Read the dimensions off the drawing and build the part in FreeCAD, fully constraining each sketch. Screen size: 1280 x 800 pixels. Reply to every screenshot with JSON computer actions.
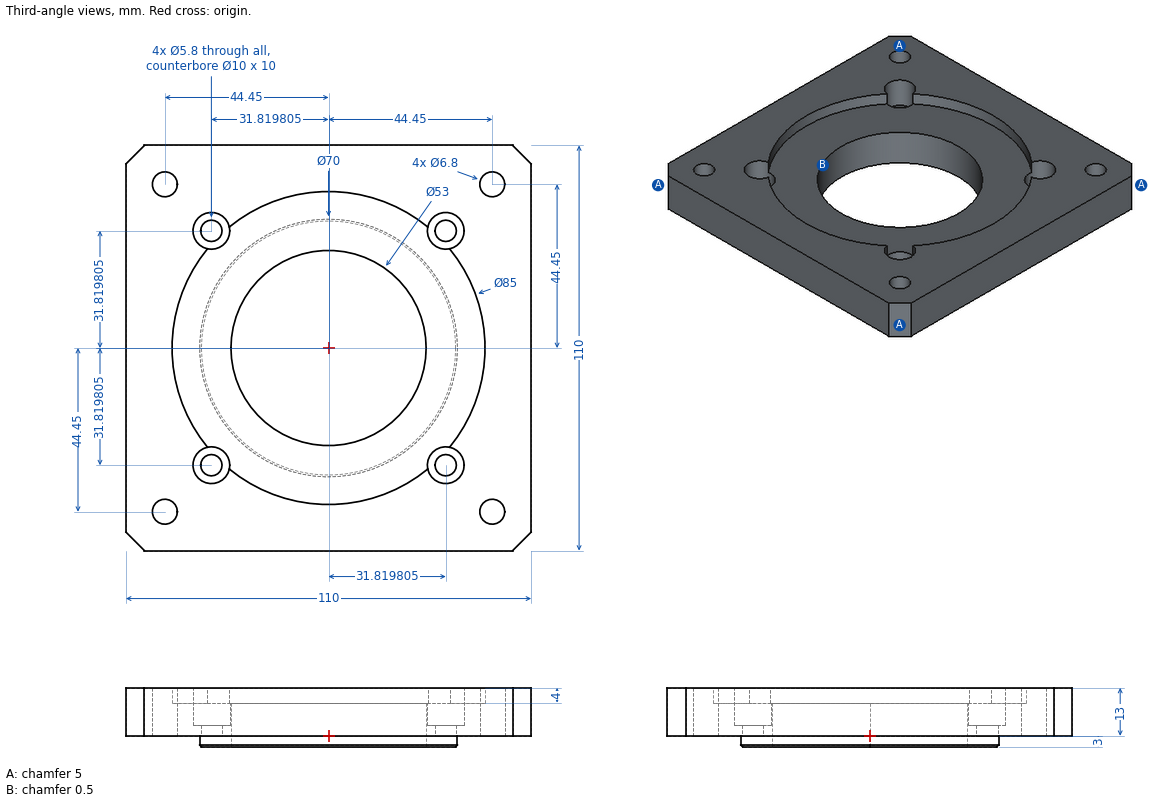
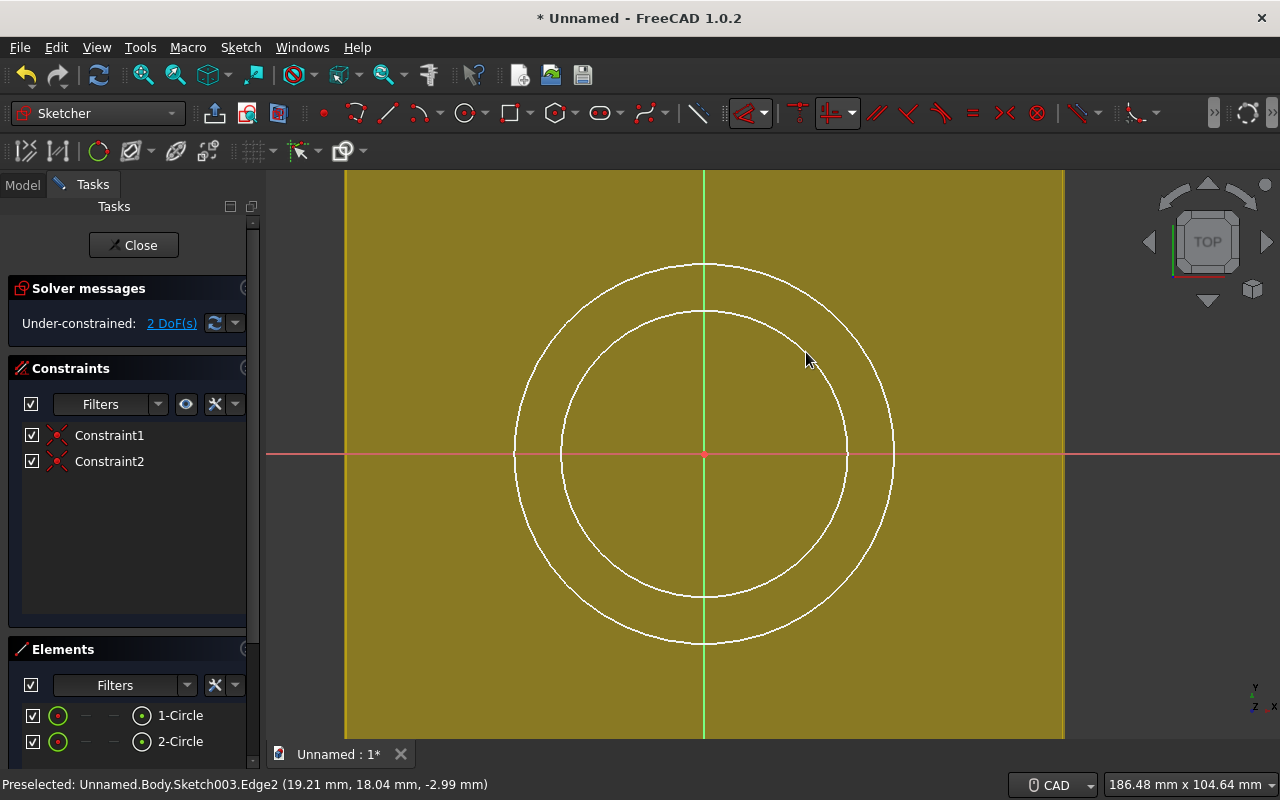
{"action": "left_click", "coordinate": [838, 319]}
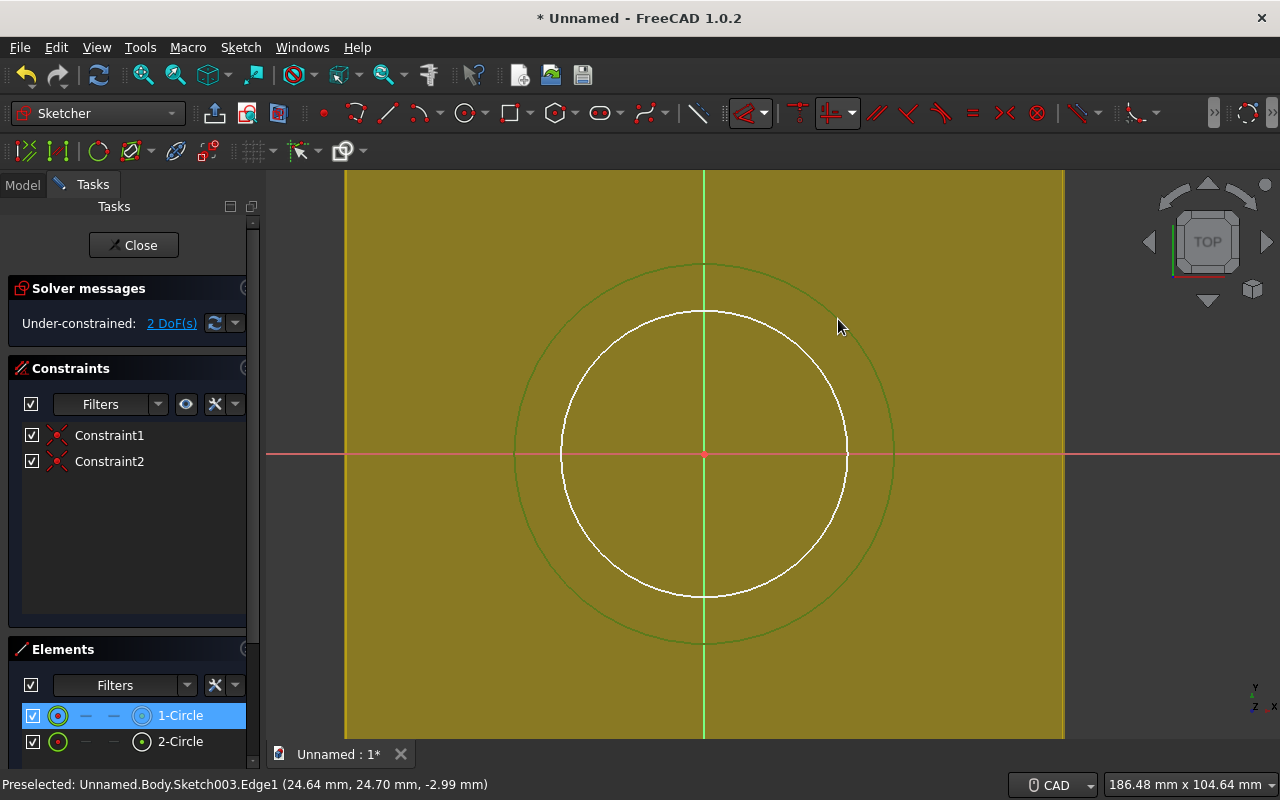
{"action": "left_click", "coordinate": [766, 114]}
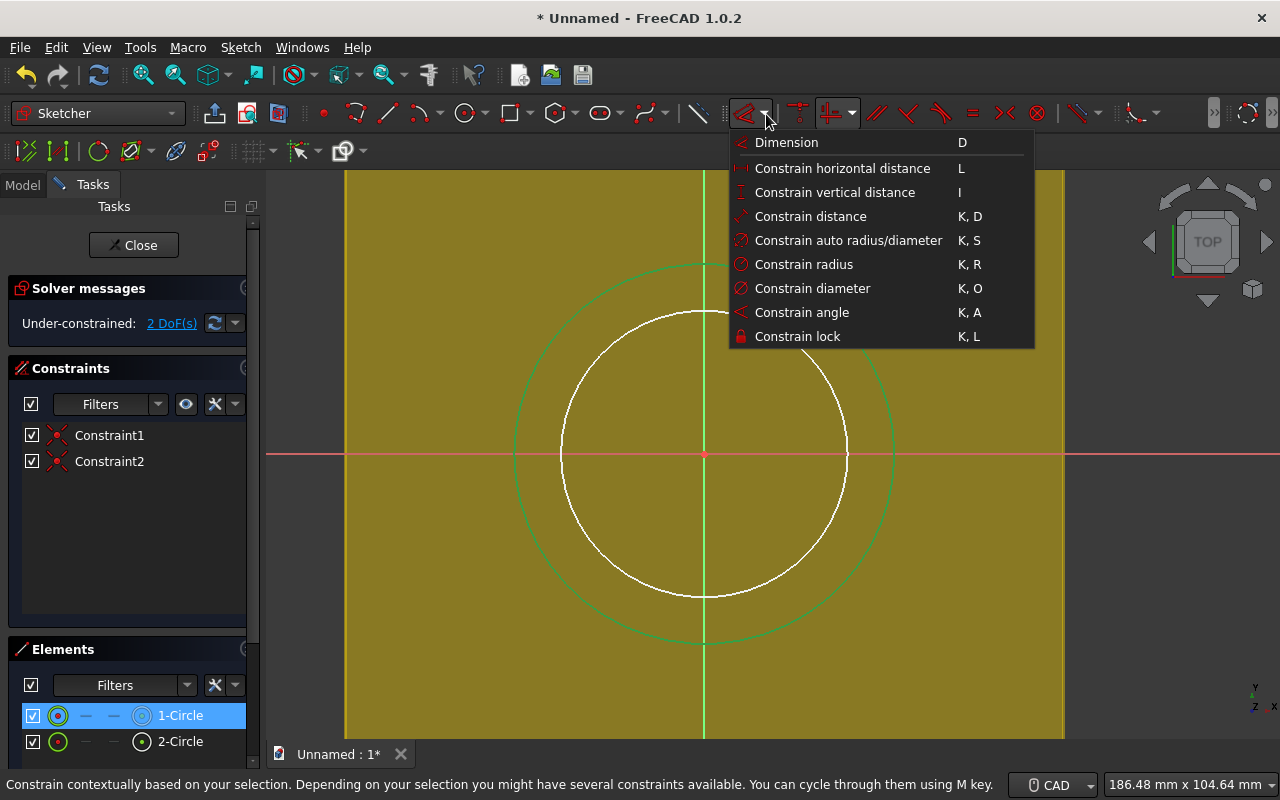
{"action": "left_click", "coordinate": [882, 288]}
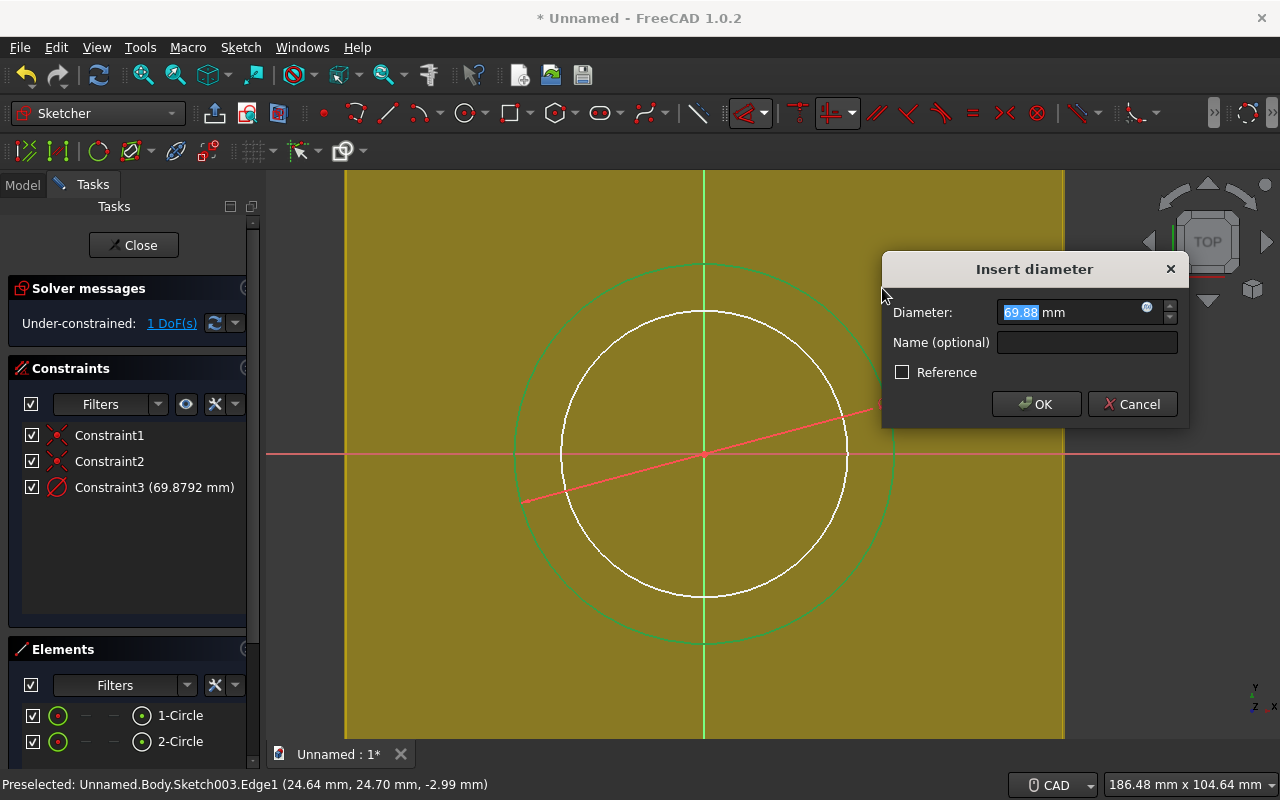
{"action": "type", "text": "70"}
{"action": "key", "text": "Return"}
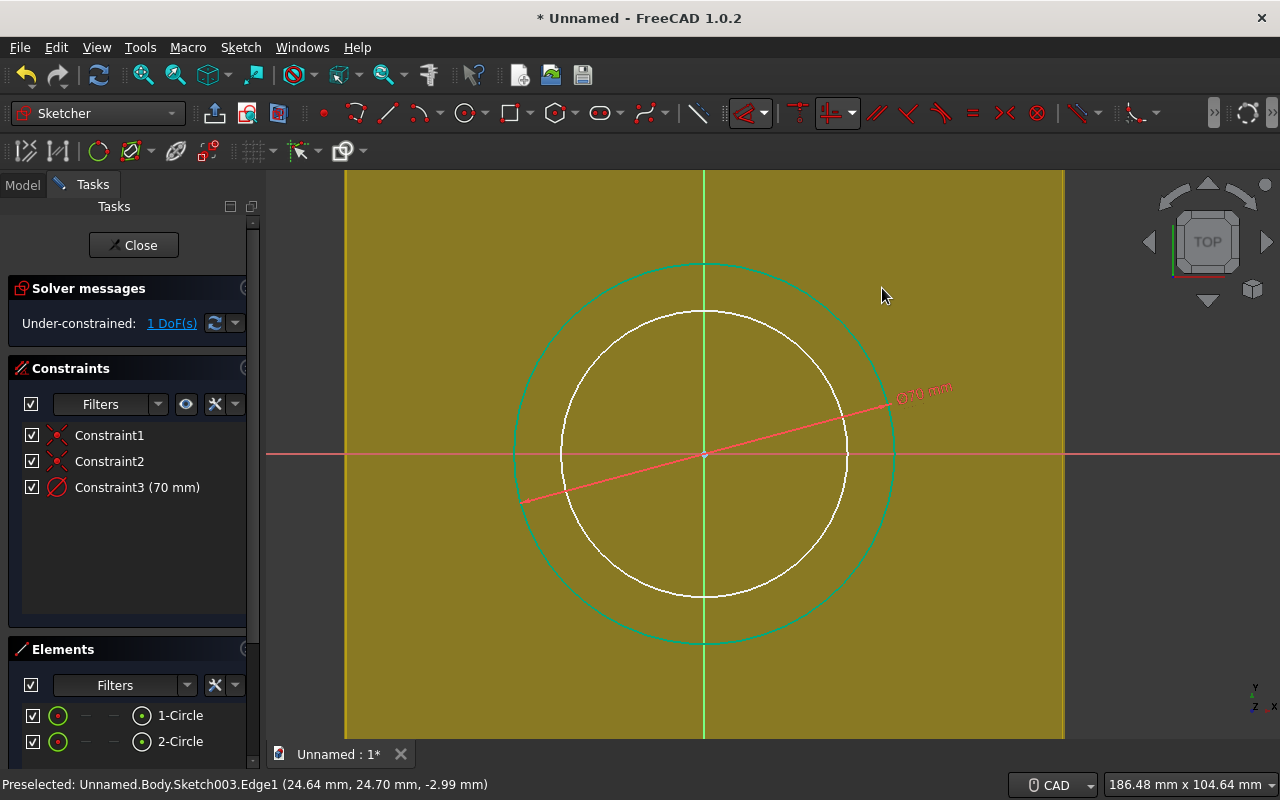
{"action": "left_click", "coordinate": [805, 352]}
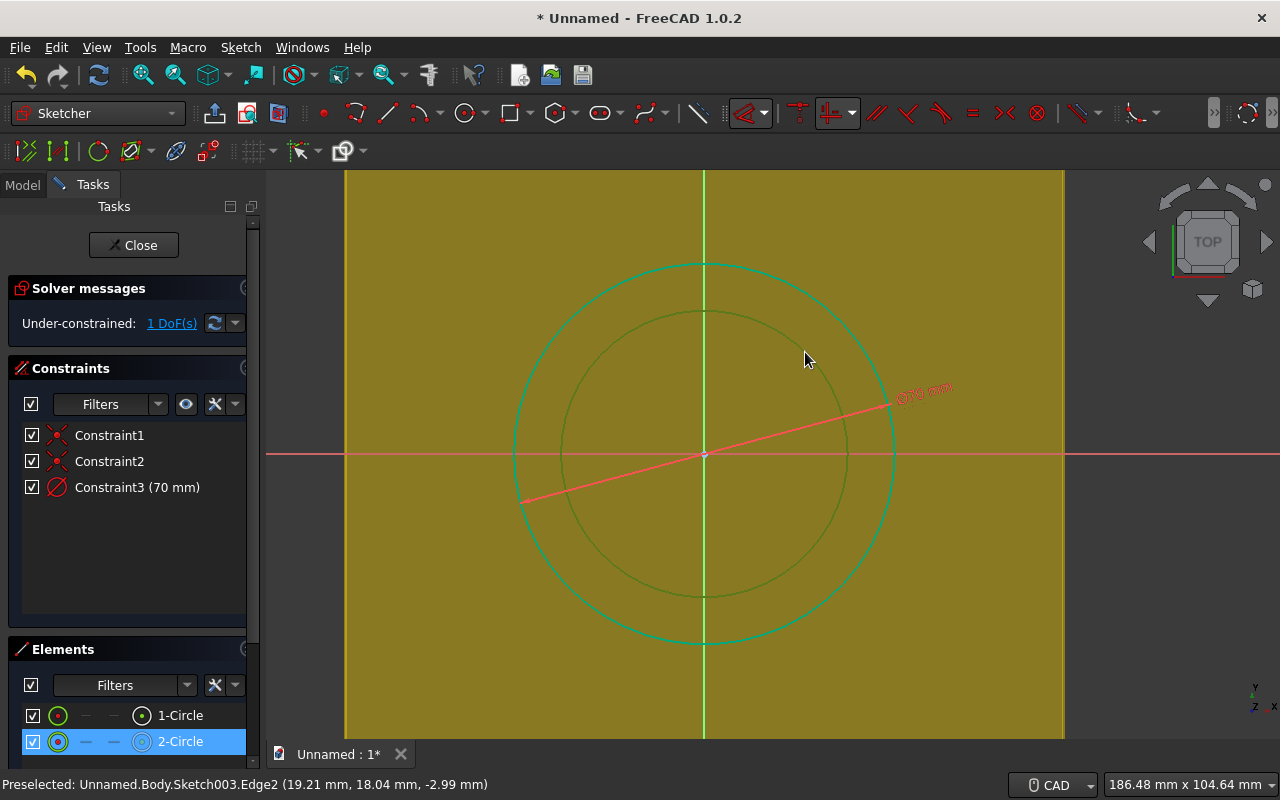
{"action": "key", "text": "k o"}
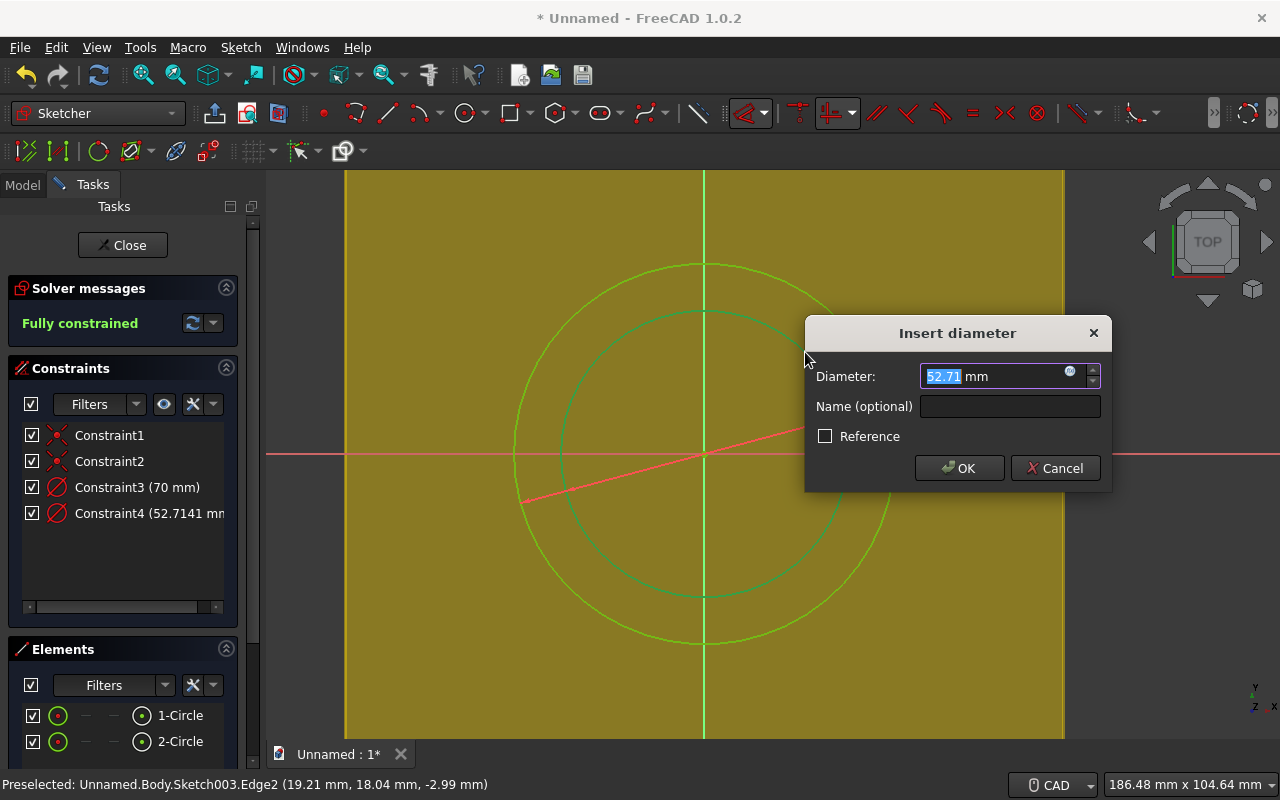
{"action": "type", "text": "53"}
{"action": "key", "text": "Return"}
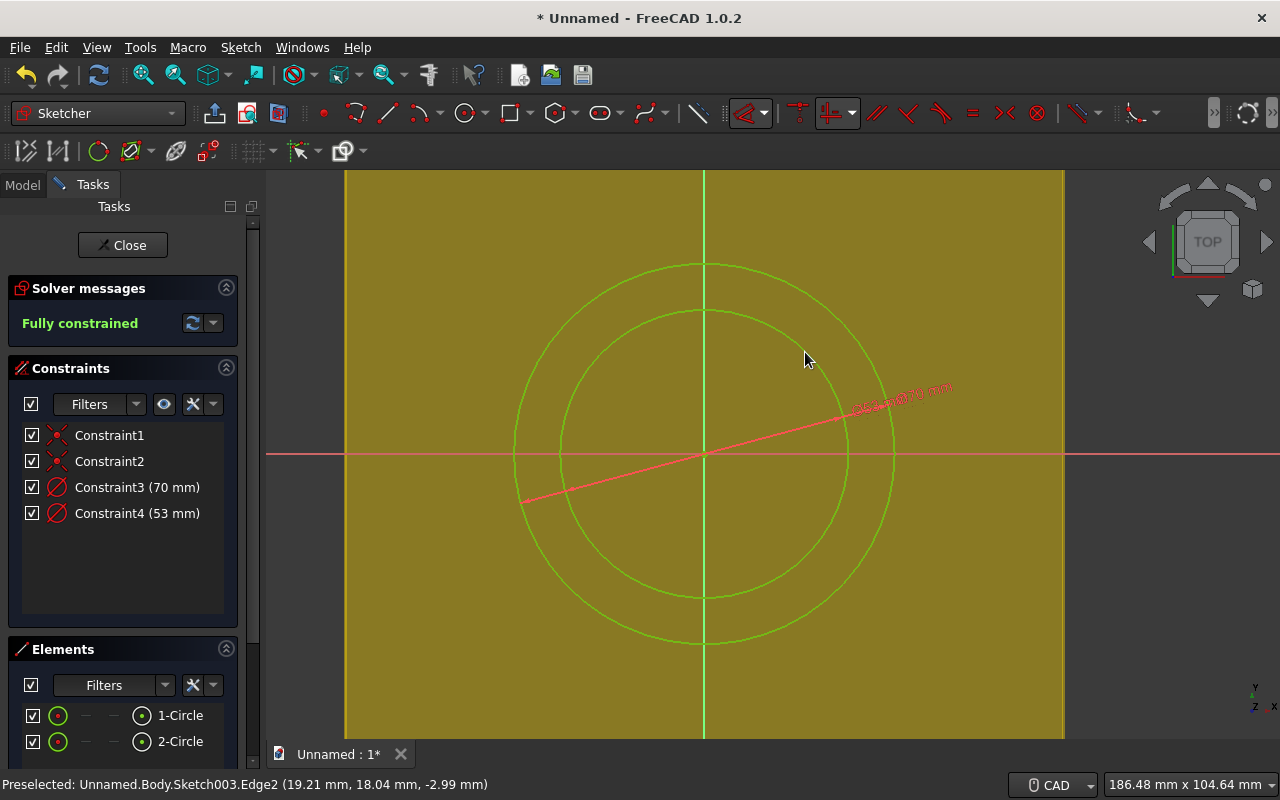
{"action": "left_click", "coordinate": [123, 245]}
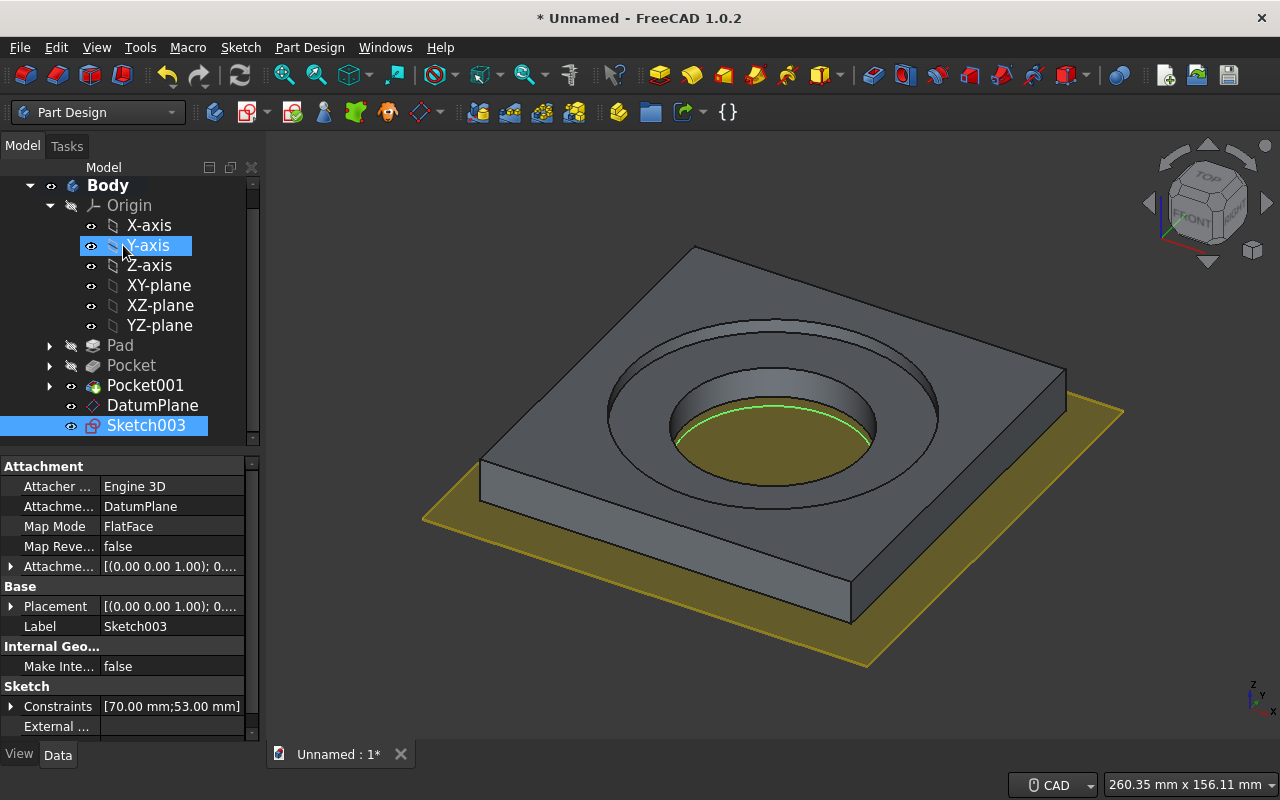
{"action": "left_click", "coordinate": [660, 76]}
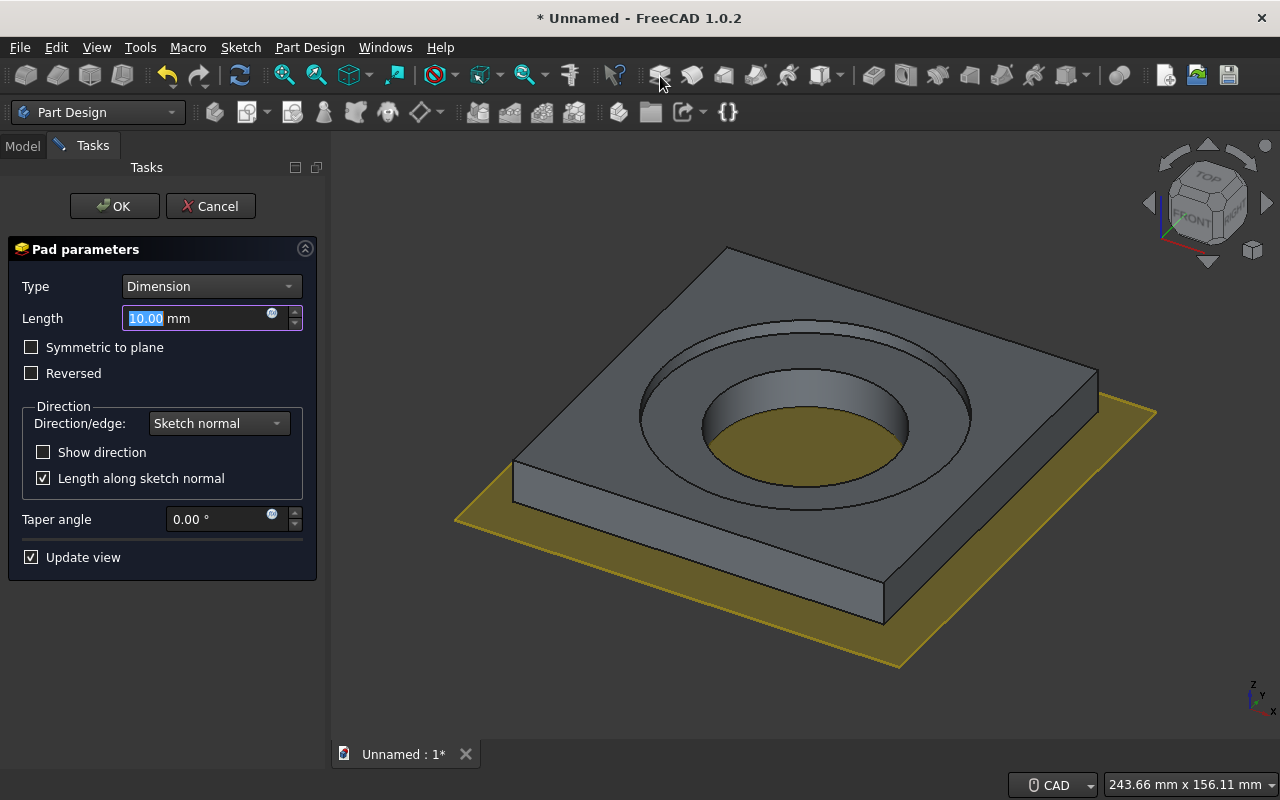
{"action": "type", "text": "3"}
{"action": "key", "text": "Tab"}